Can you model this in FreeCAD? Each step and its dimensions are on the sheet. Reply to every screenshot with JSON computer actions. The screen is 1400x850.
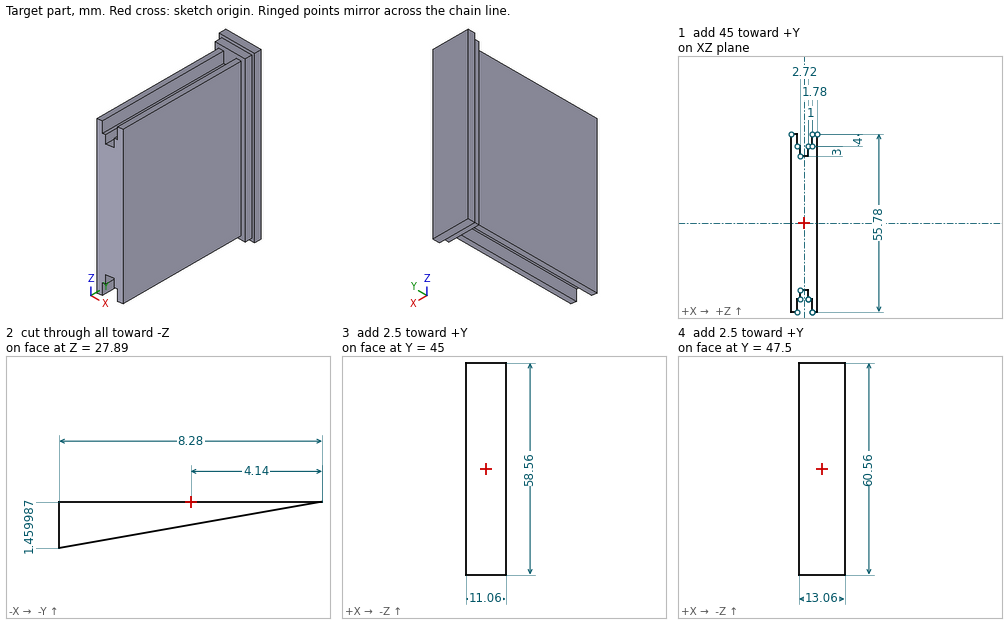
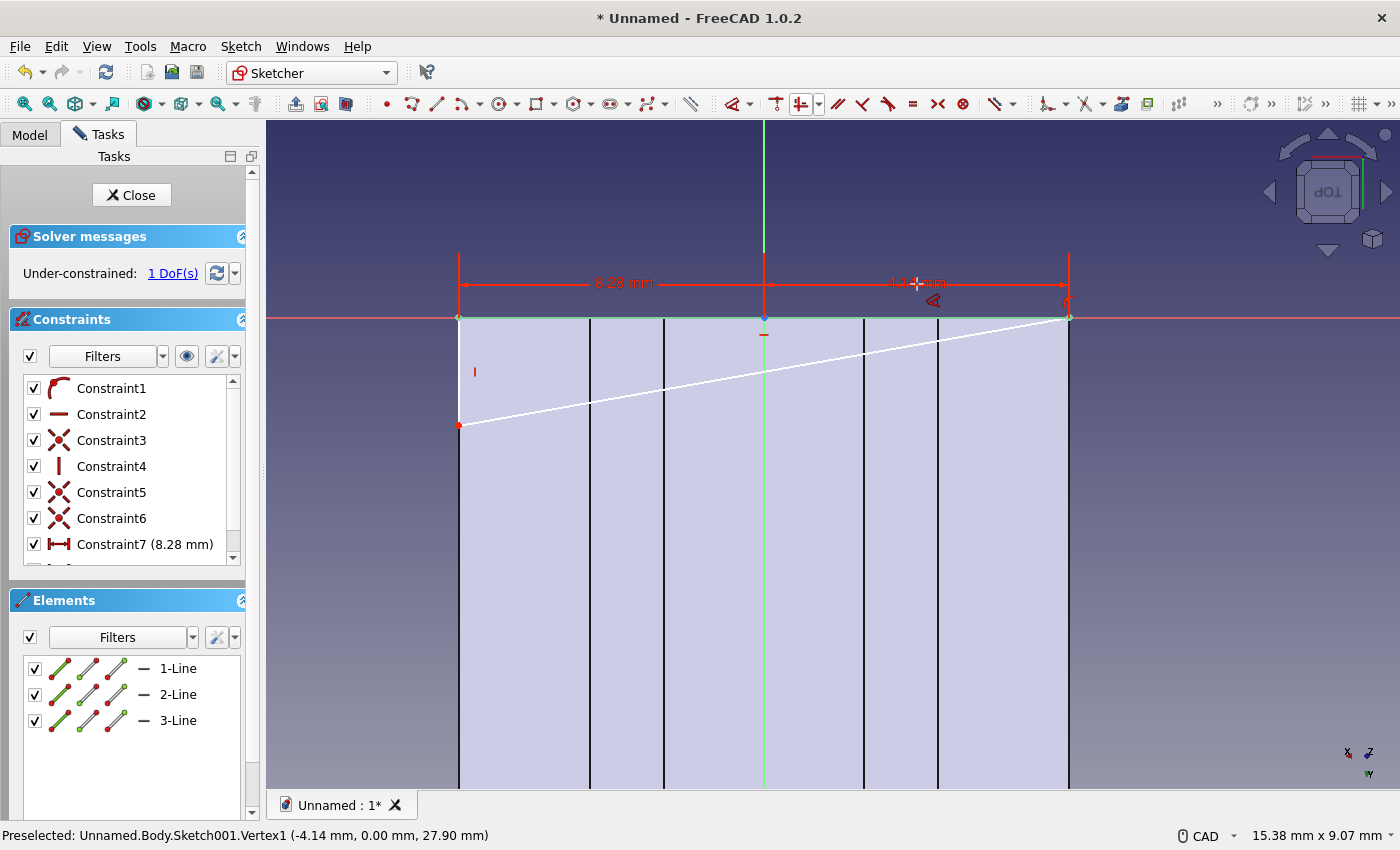
{"action": "left_click", "coordinate": [459, 350]}
{"action": "left_click", "coordinate": [425, 372]}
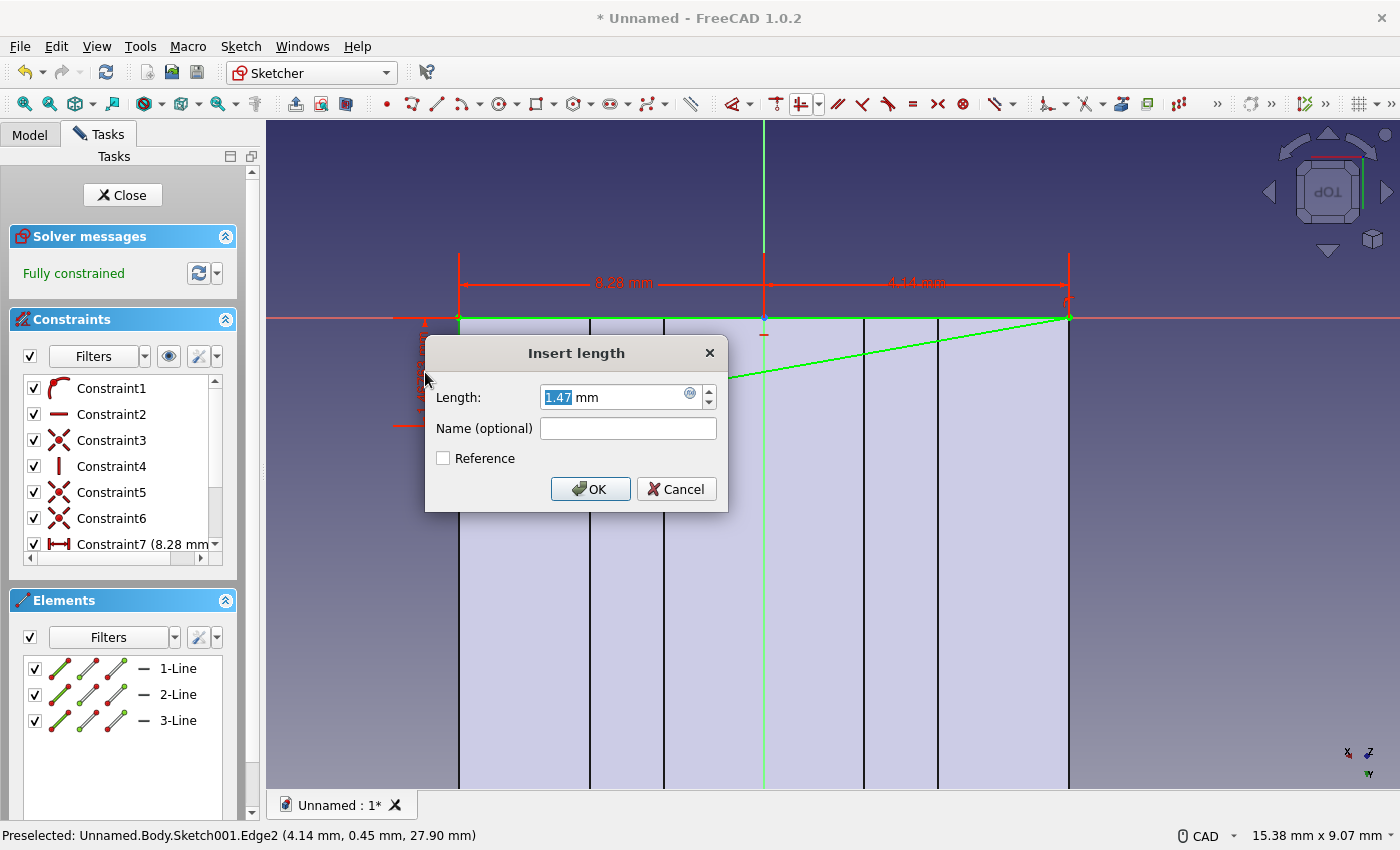
{"action": "type", "text": "1.459987"}
{"action": "key", "text": "Return"}
{"action": "key", "text": "Escape"}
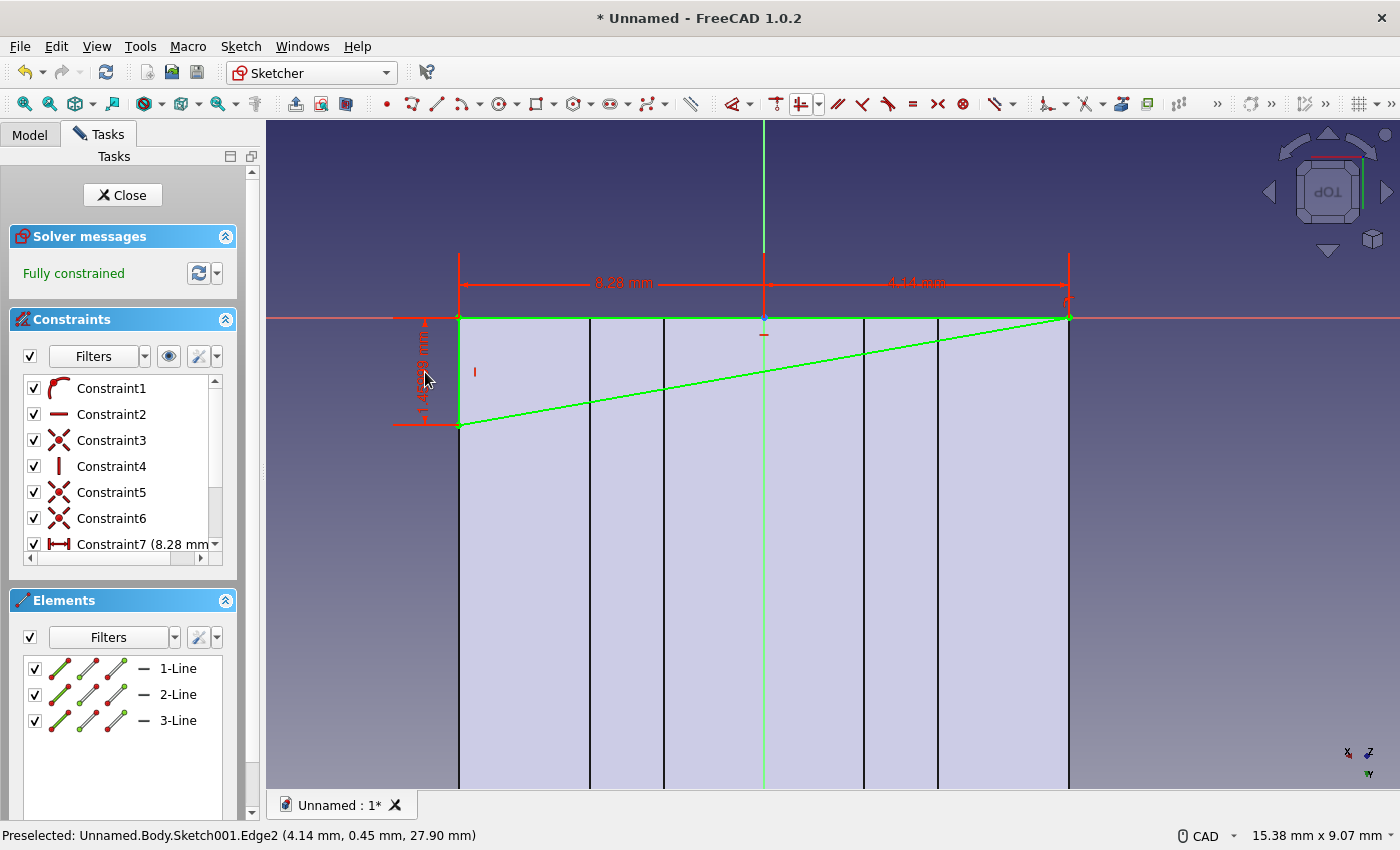
{"action": "left_click", "coordinate": [123, 195]}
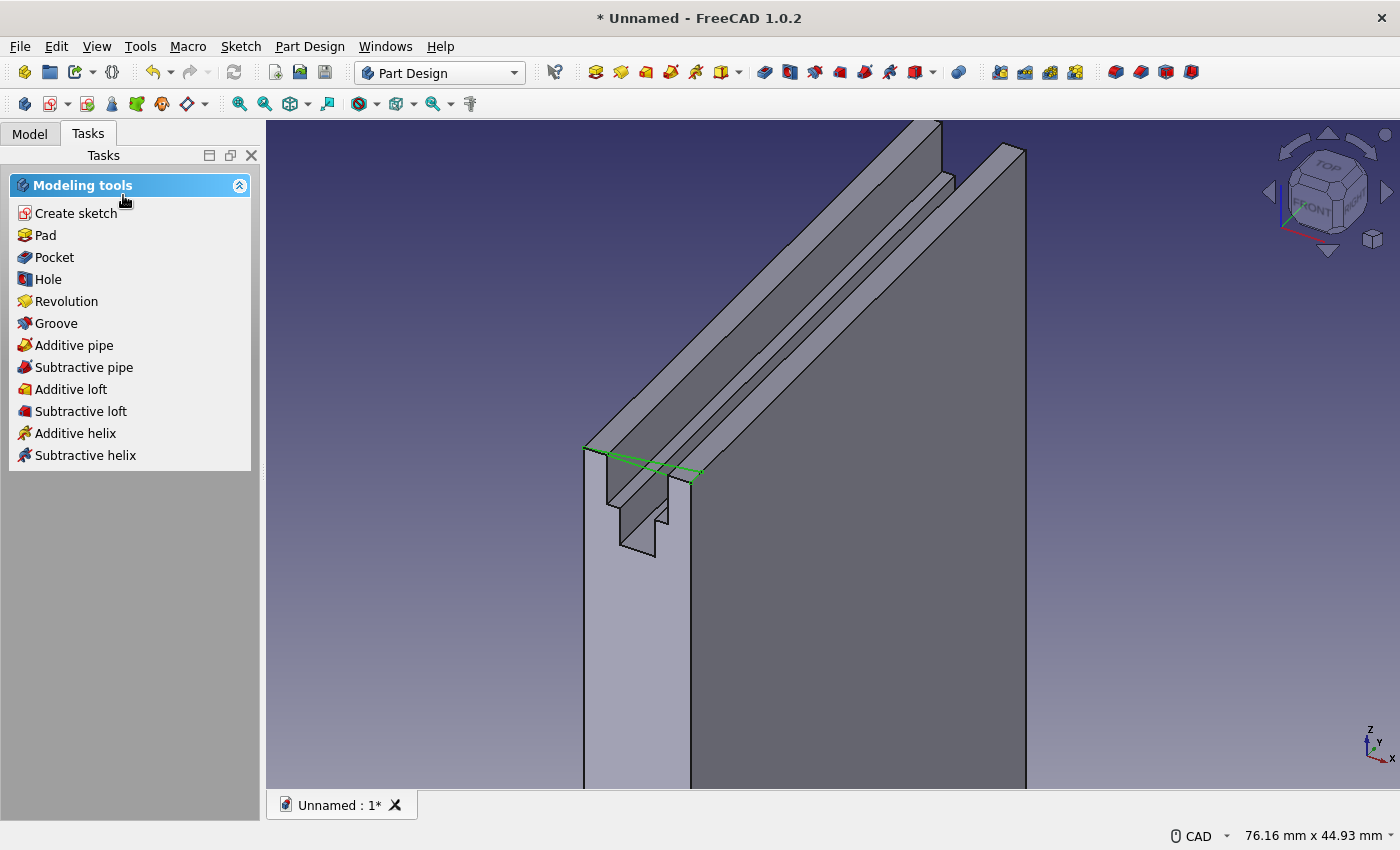
{"action": "left_click", "coordinate": [765, 72]}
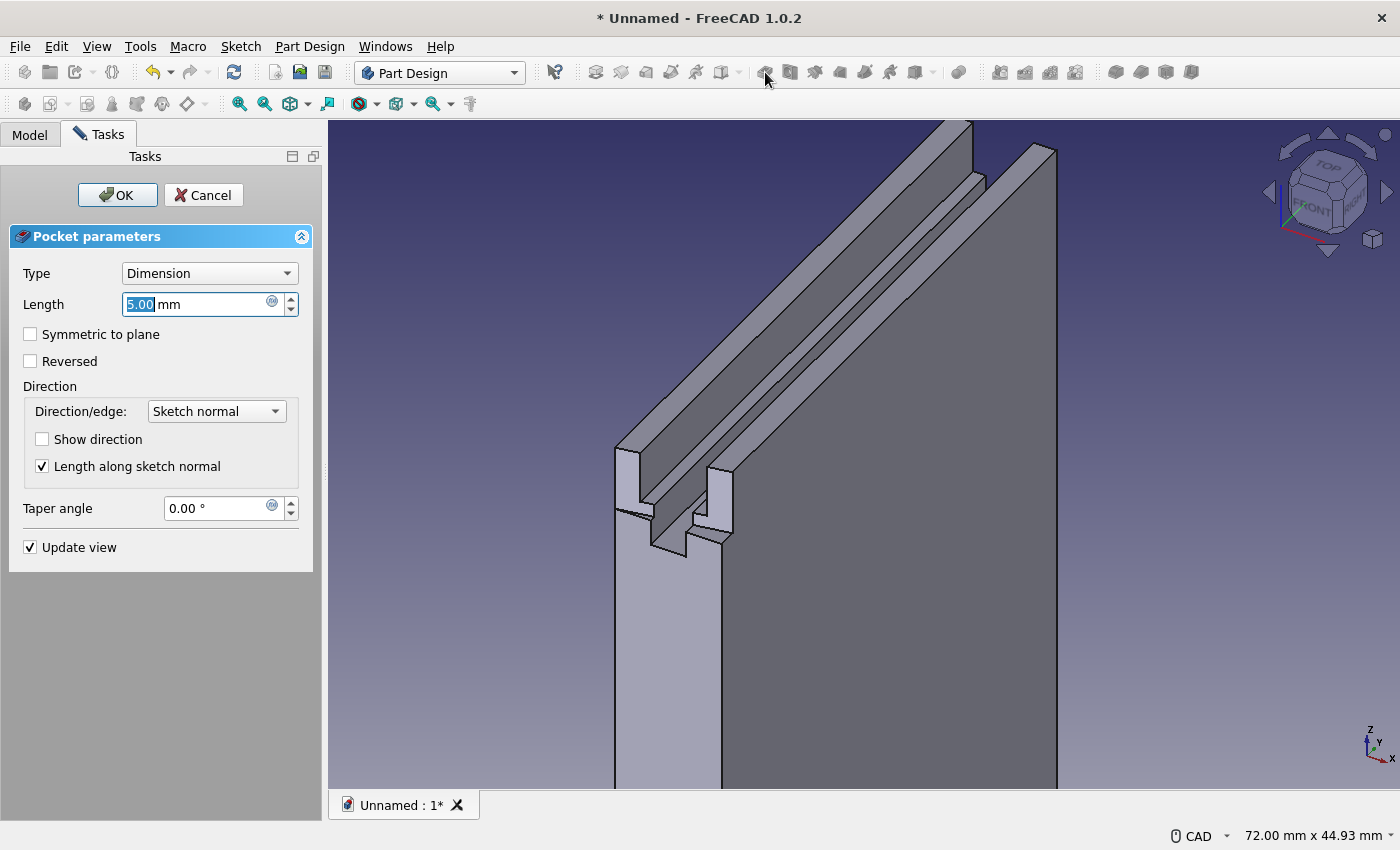
{"action": "left_click", "coordinate": [210, 274]}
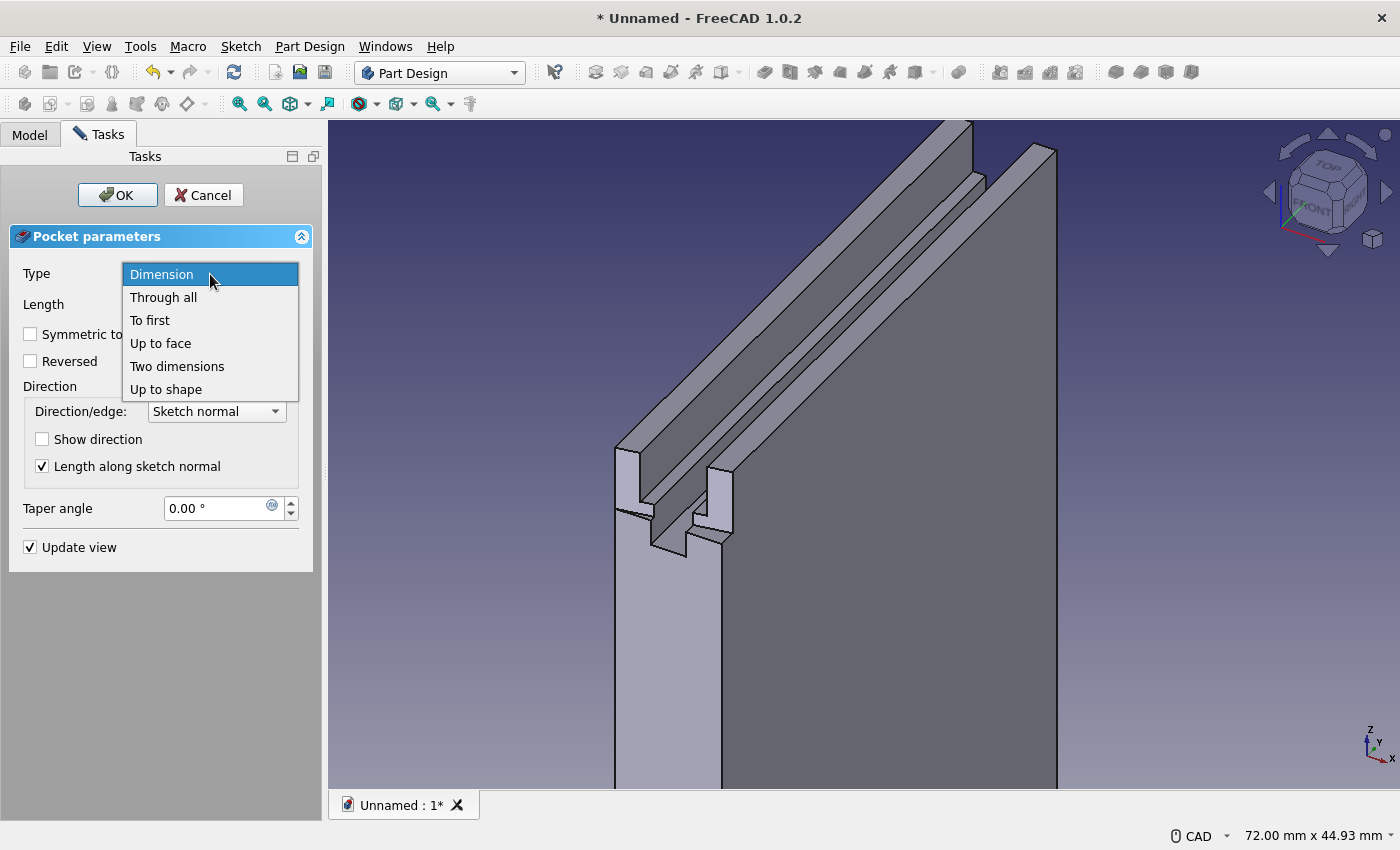
{"action": "left_click", "coordinate": [208, 298]}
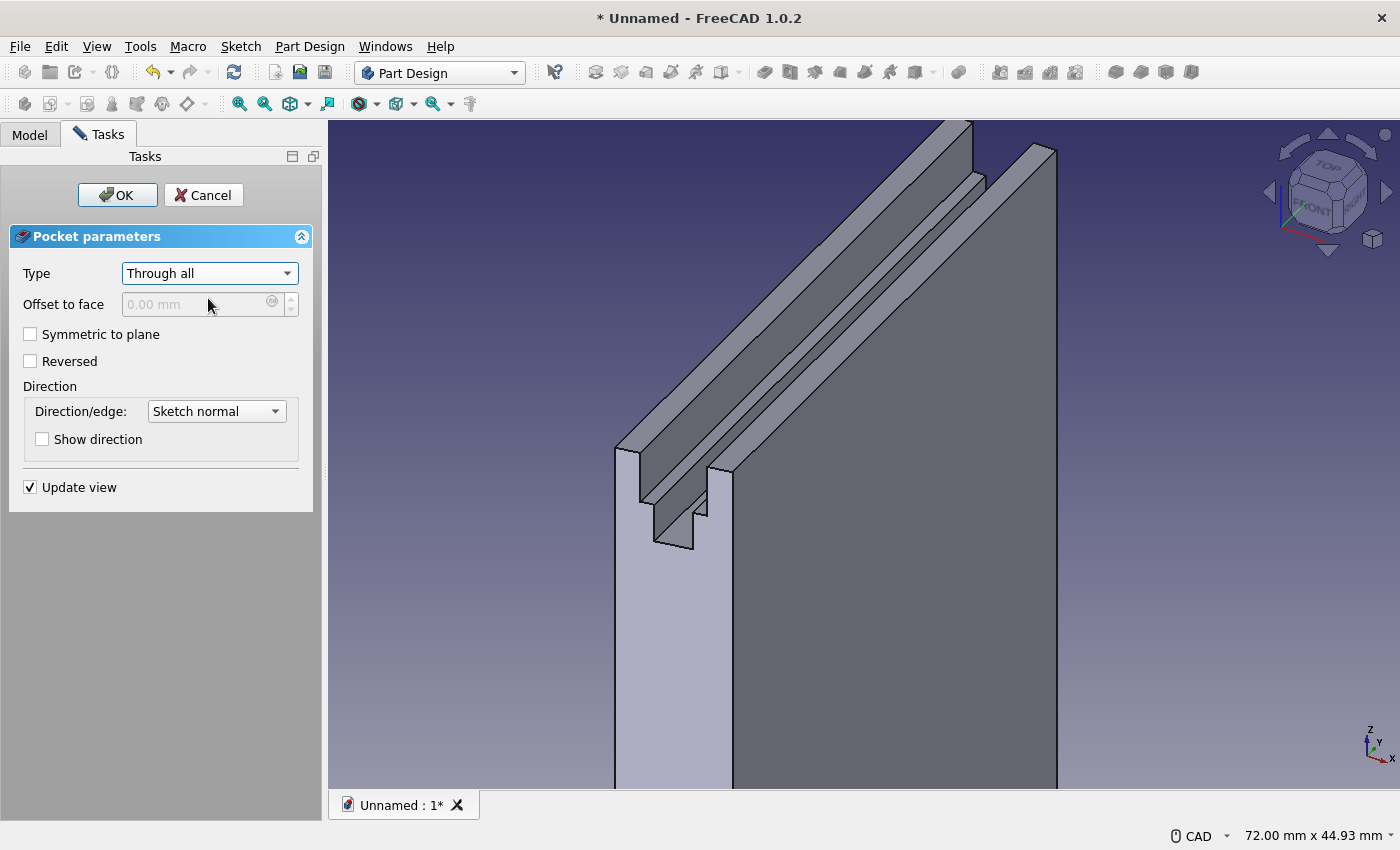
{"action": "left_click", "coordinate": [118, 195]}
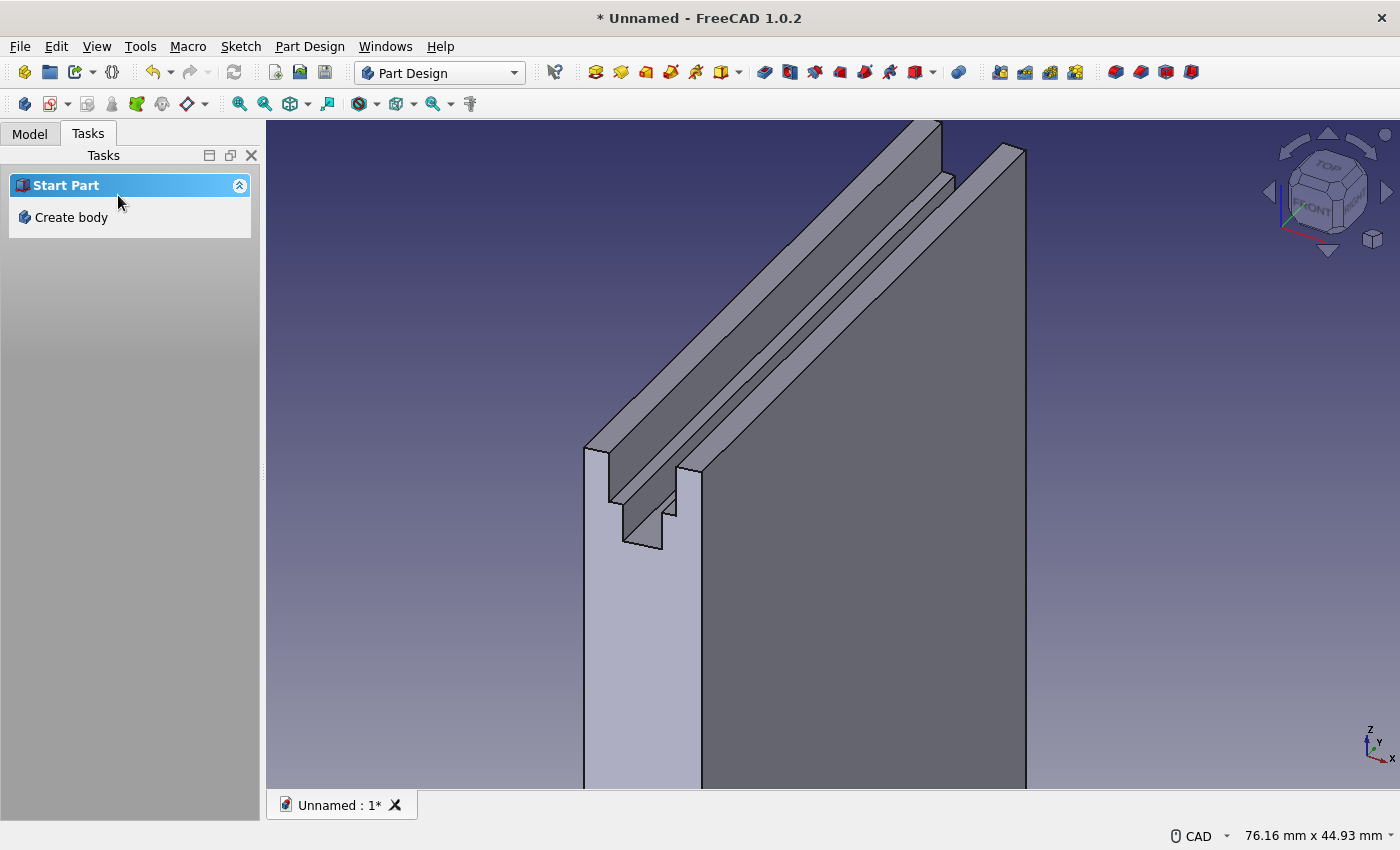
{"action": "left_click", "coordinate": [240, 104]}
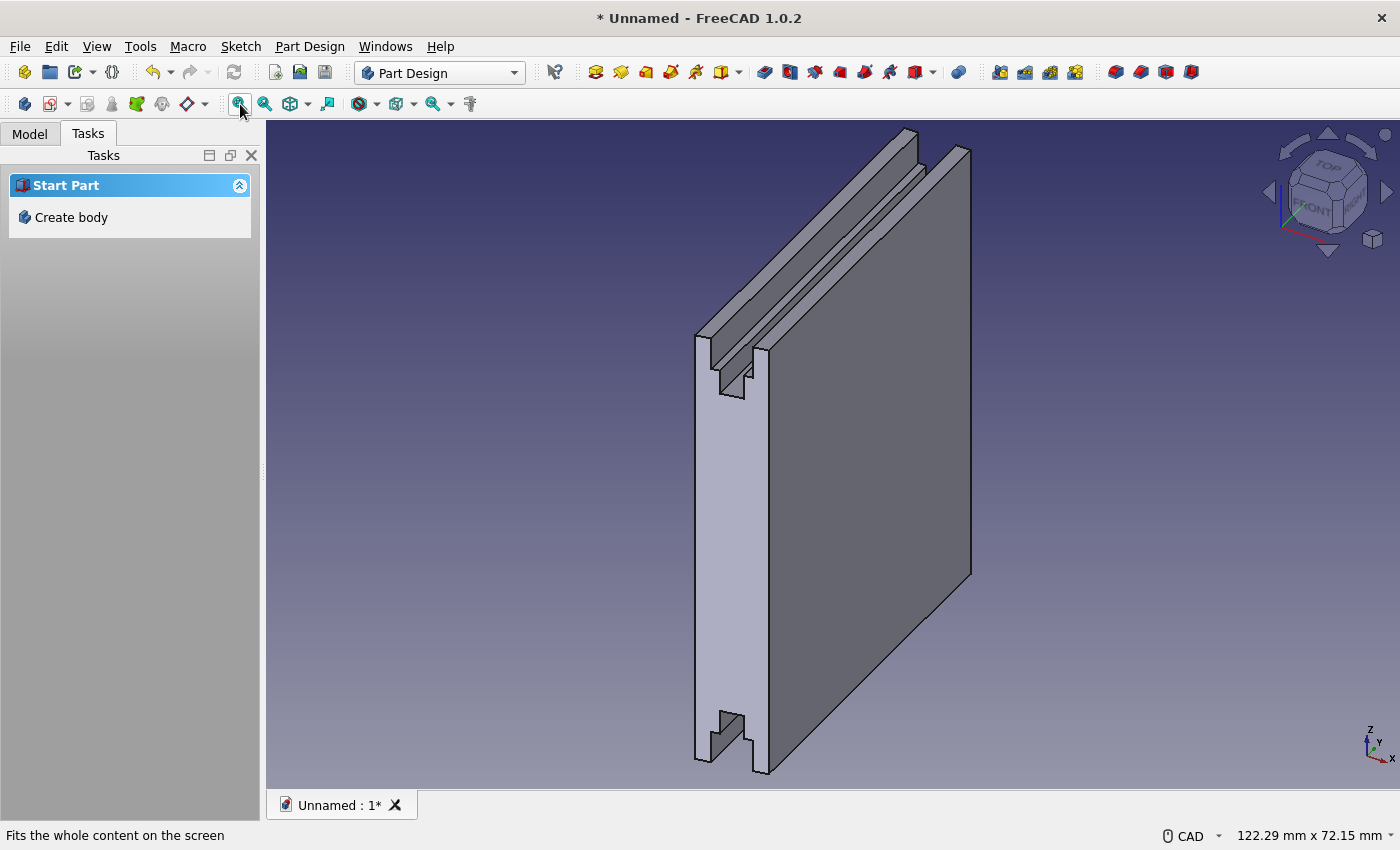
{"action": "key", "text": "4"}